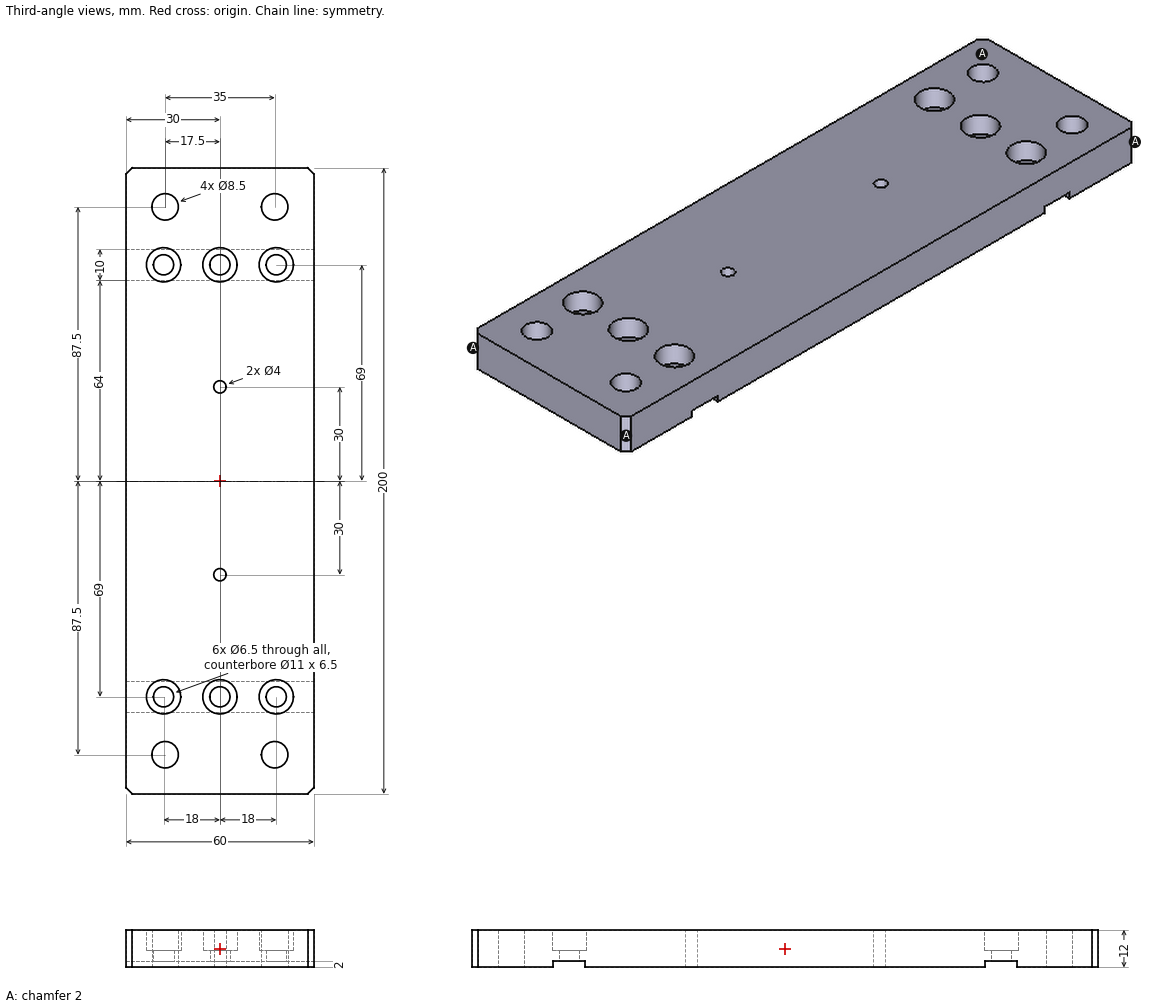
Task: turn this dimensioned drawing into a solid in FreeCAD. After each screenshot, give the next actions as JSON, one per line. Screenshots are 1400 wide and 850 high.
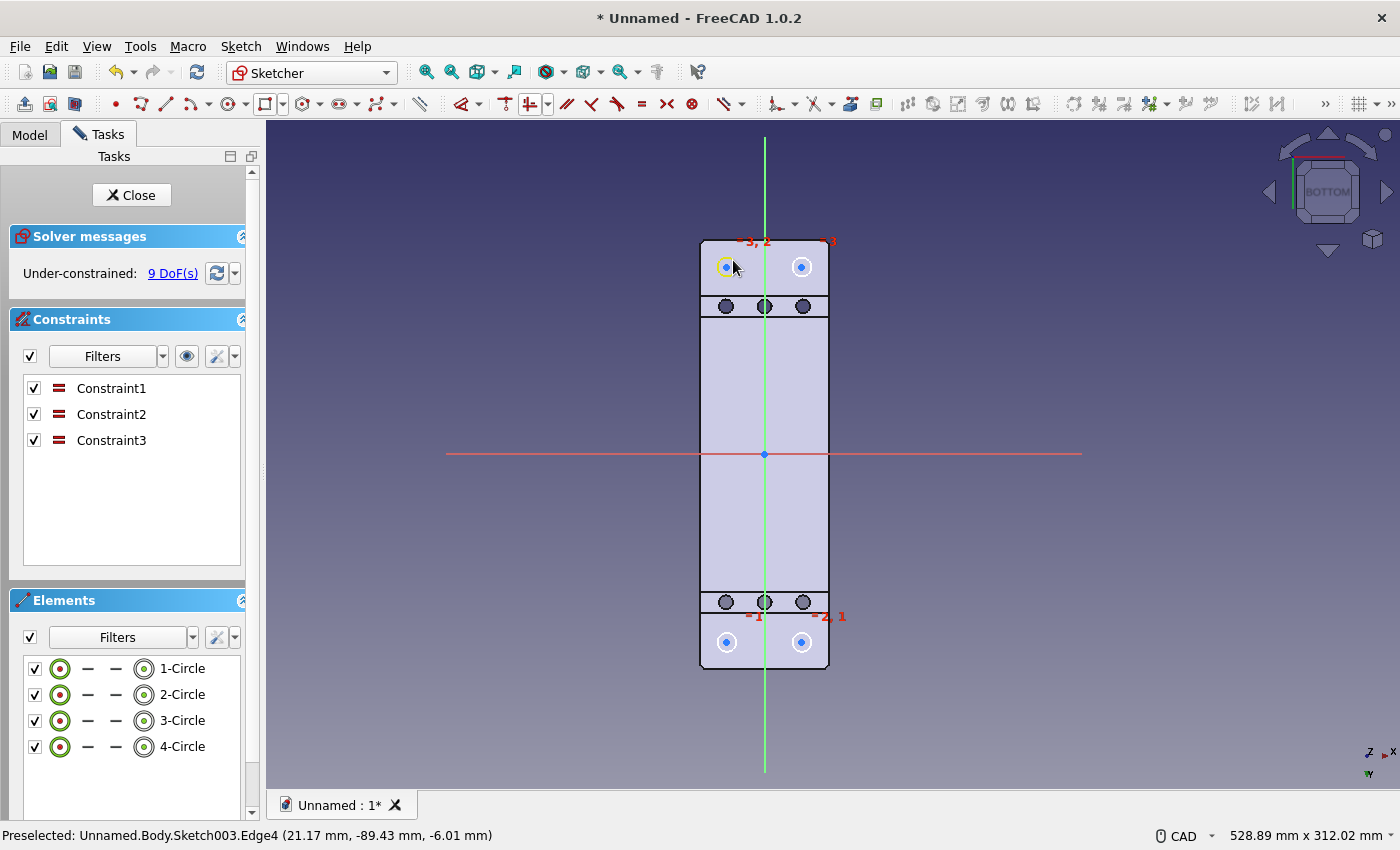
{"action": "left_click", "coordinate": [727, 642]}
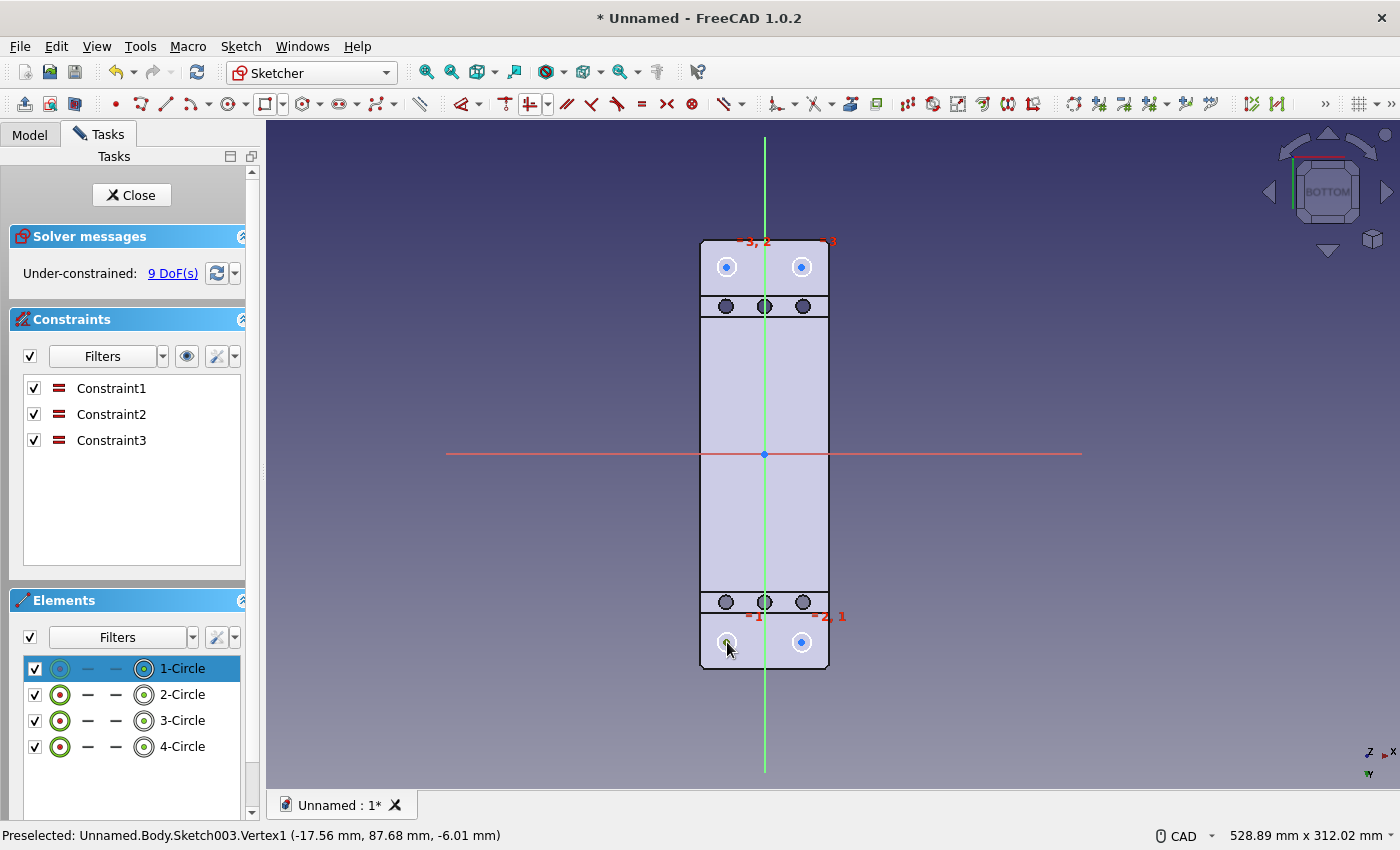
{"action": "left_click", "coordinate": [802, 642]}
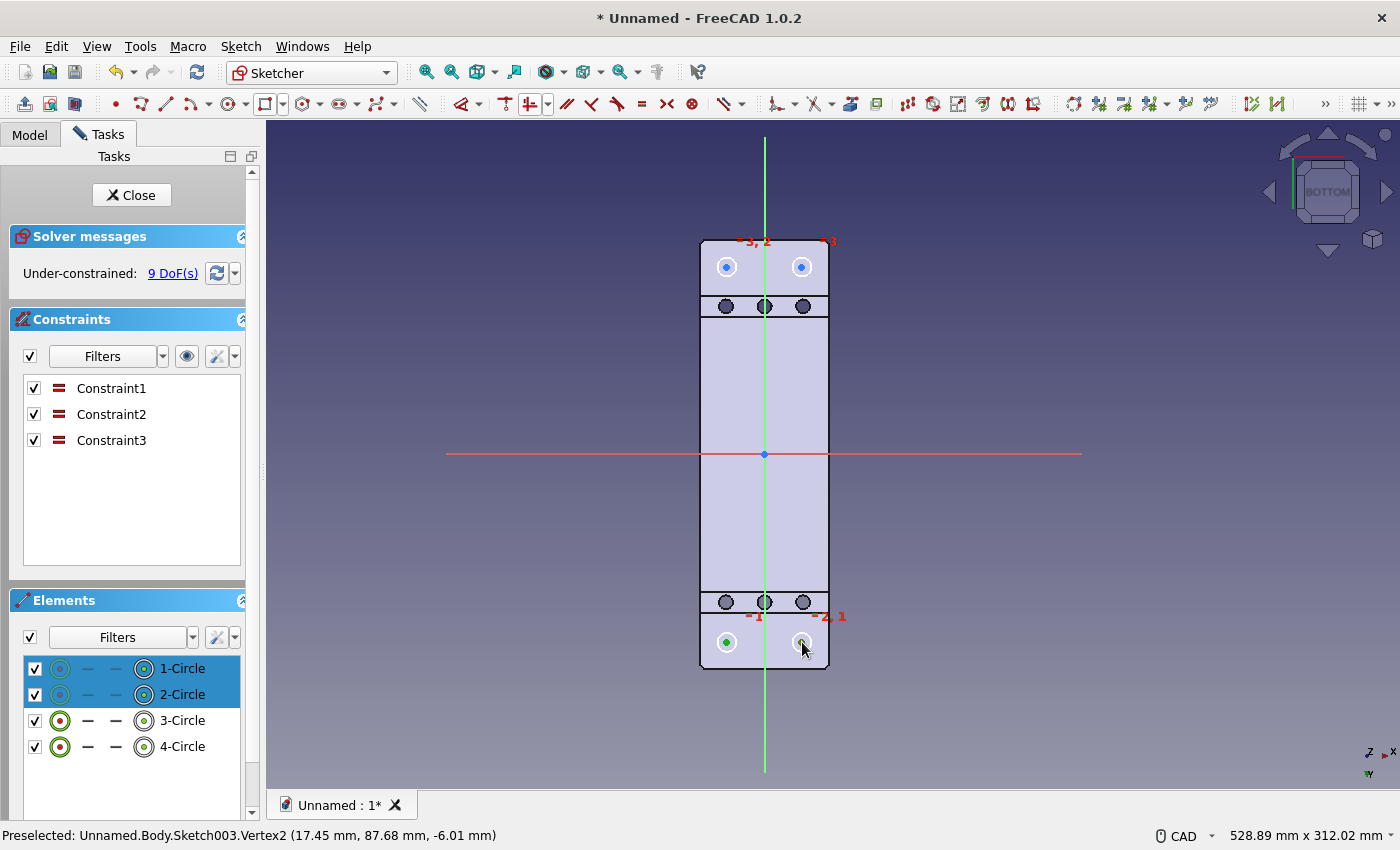
{"action": "left_click", "coordinate": [548, 104]}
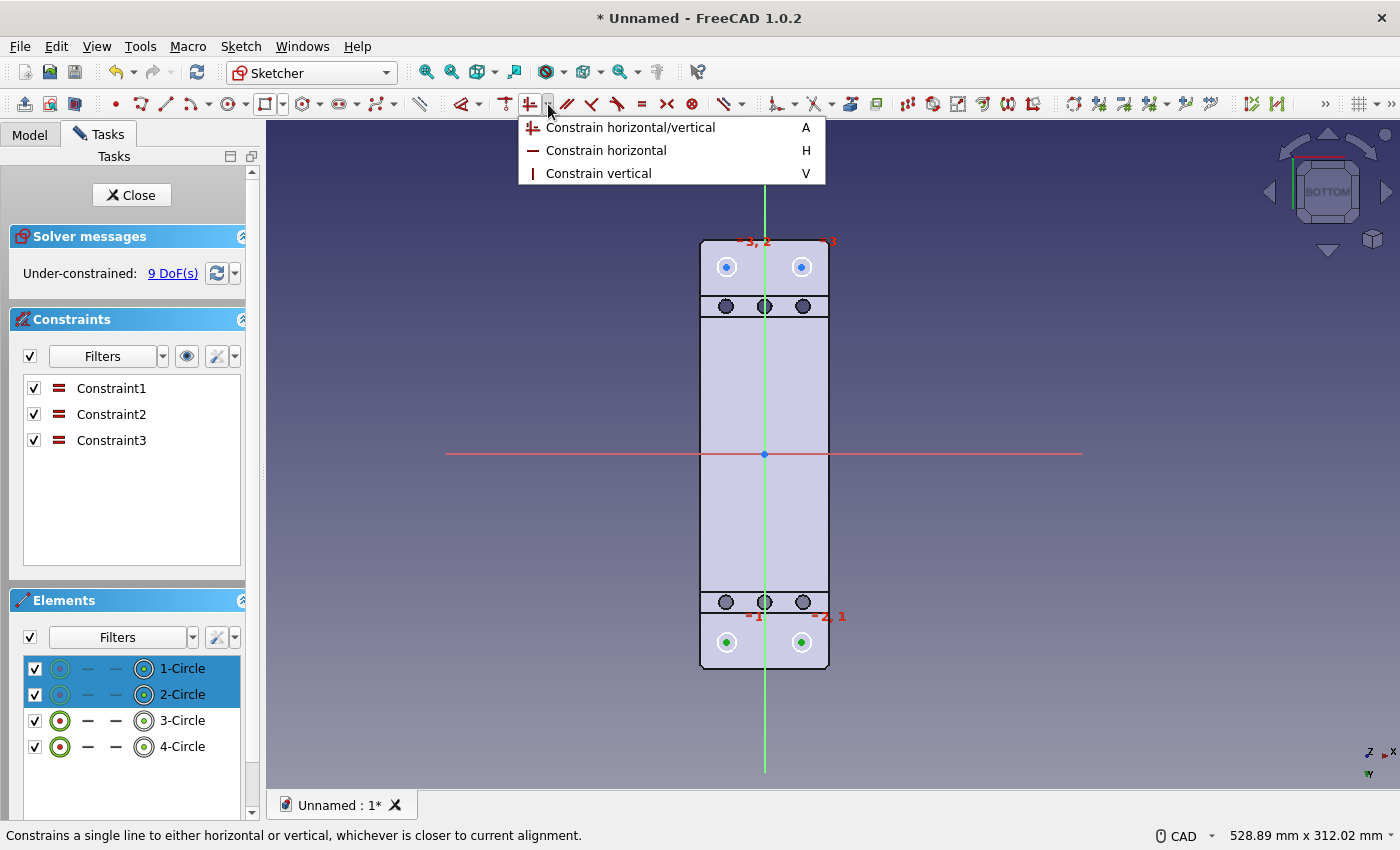
{"action": "left_click", "coordinate": [672, 150]}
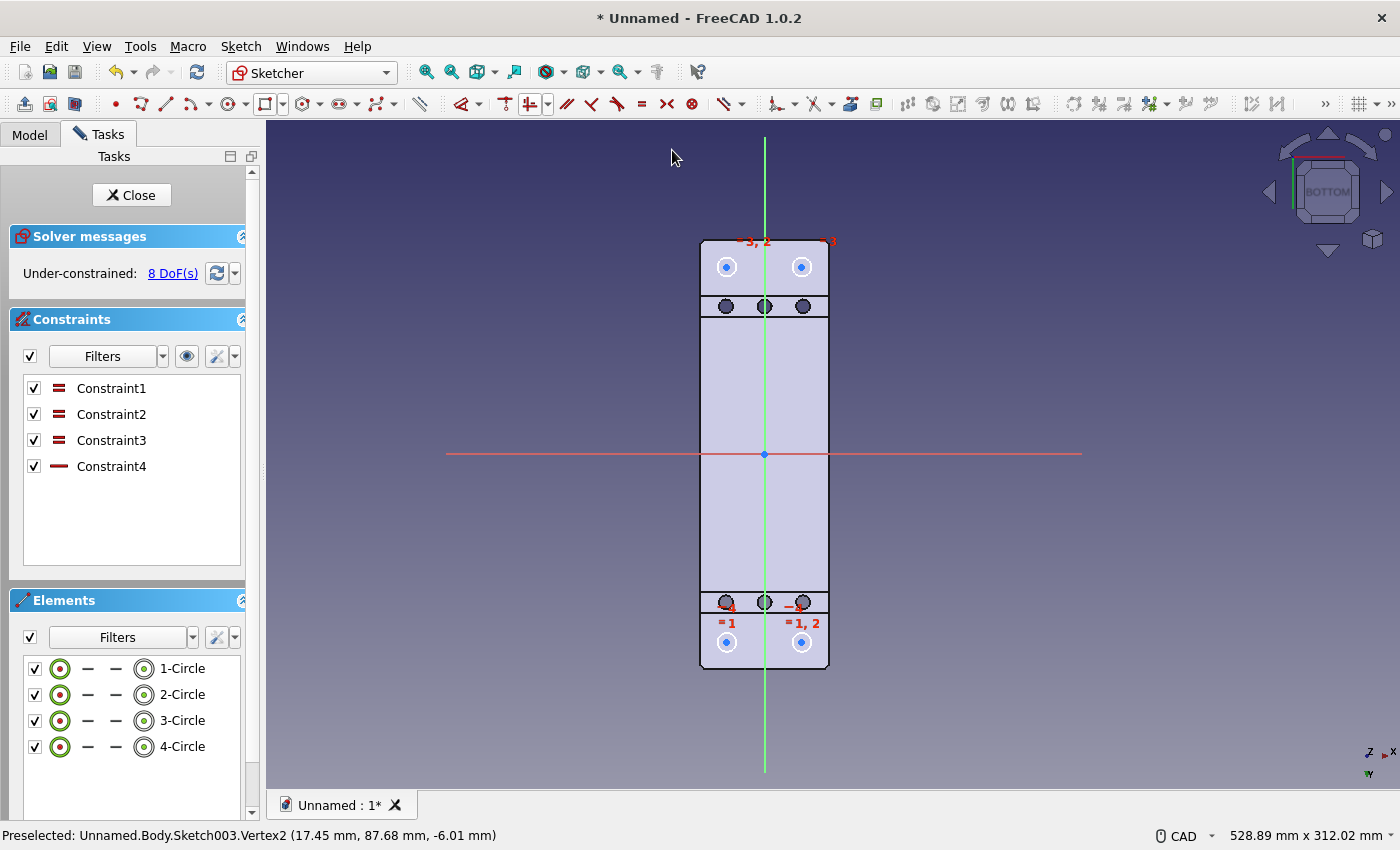
{"action": "left_click", "coordinate": [727, 642]}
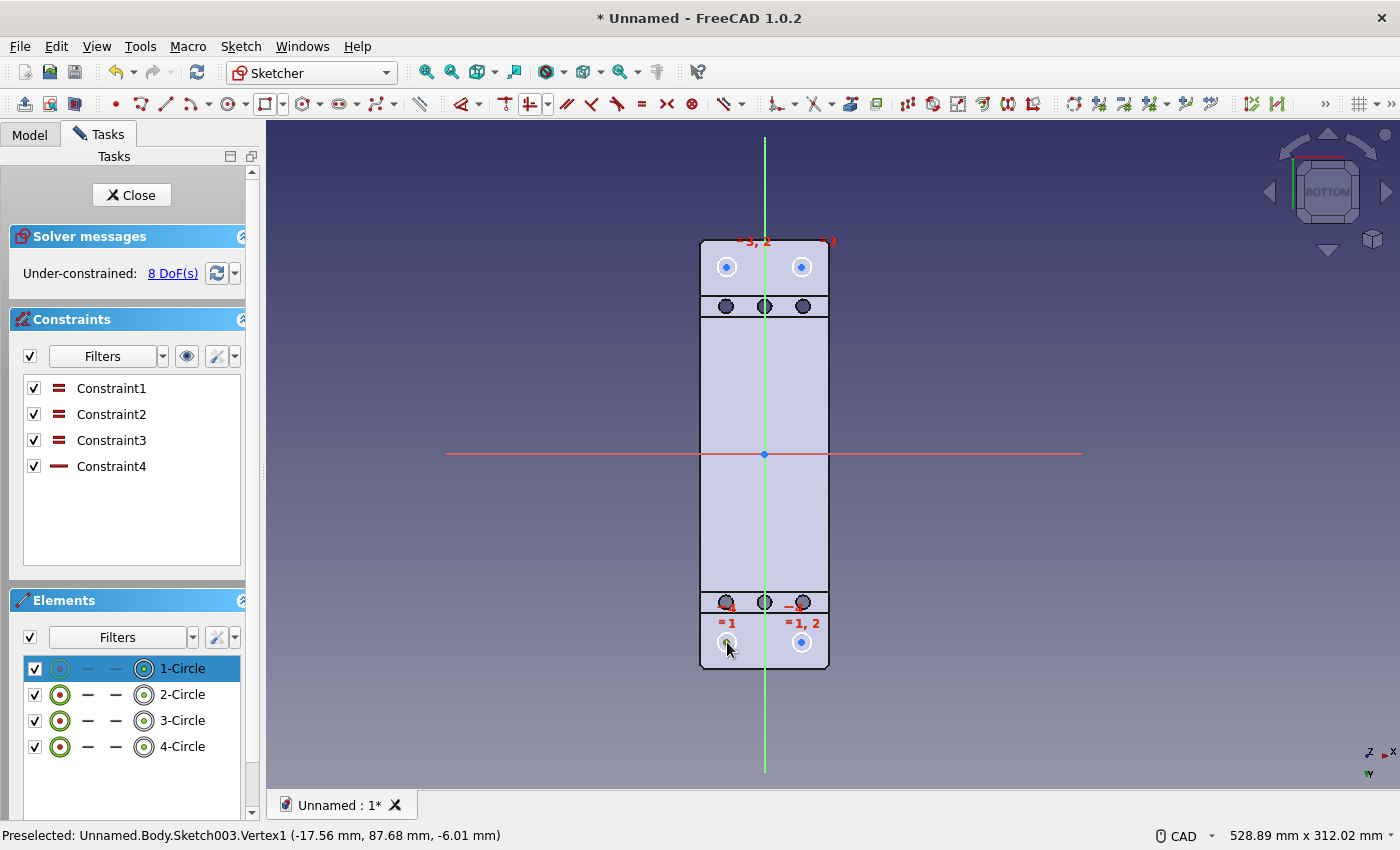
{"action": "left_click", "coordinate": [727, 267]}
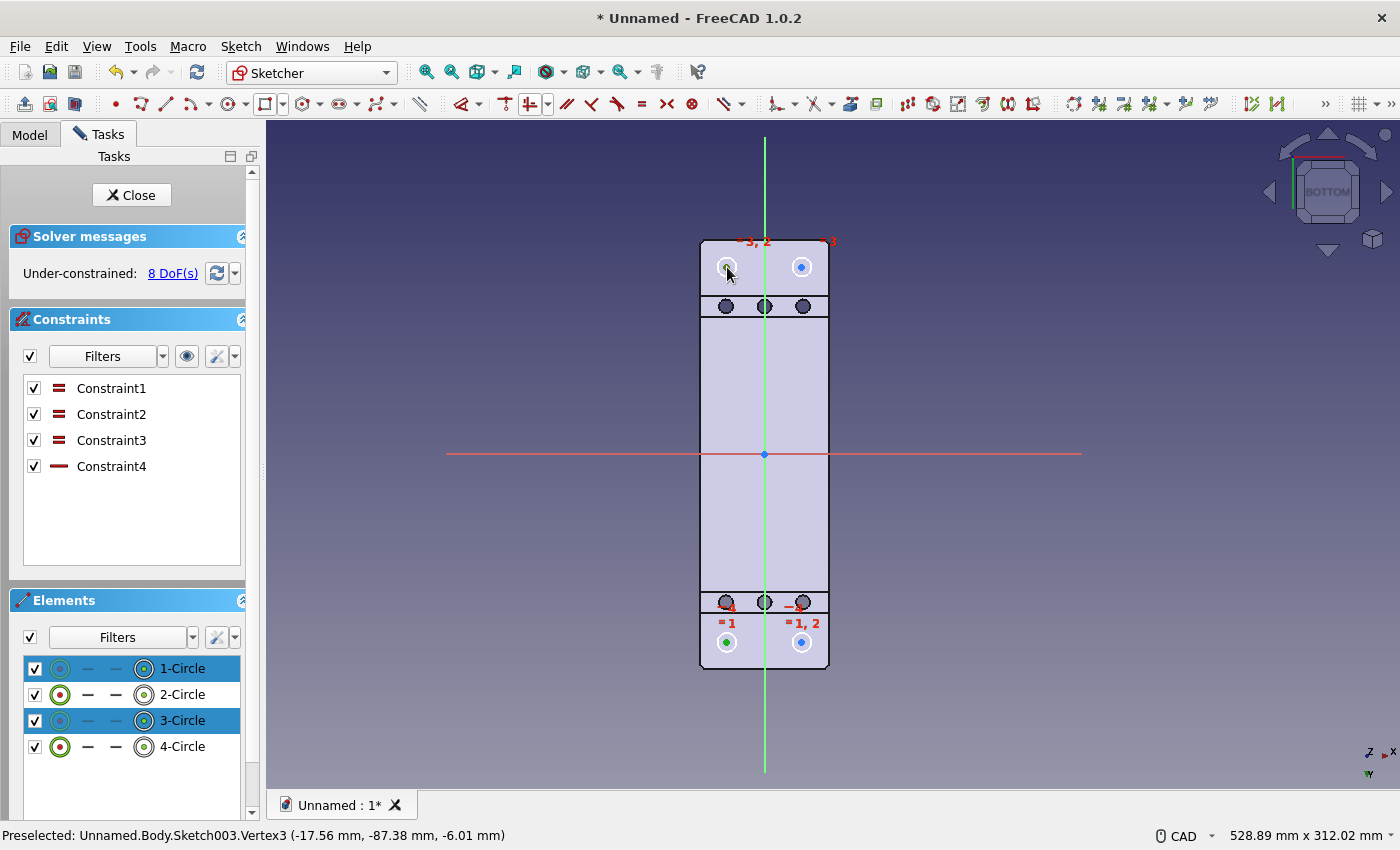
{"action": "left_click", "coordinate": [548, 104]}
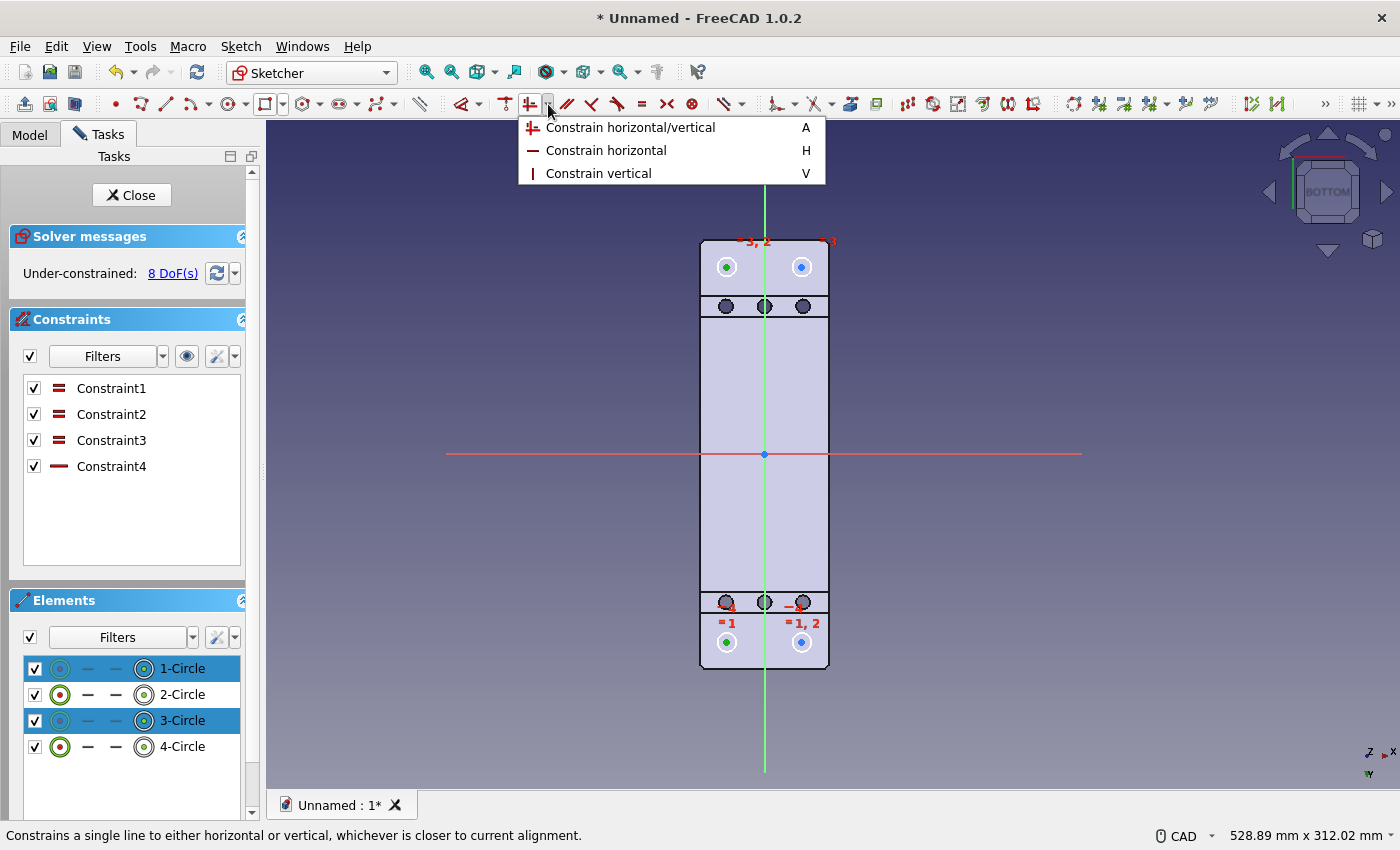
{"action": "left_click", "coordinate": [672, 174]}